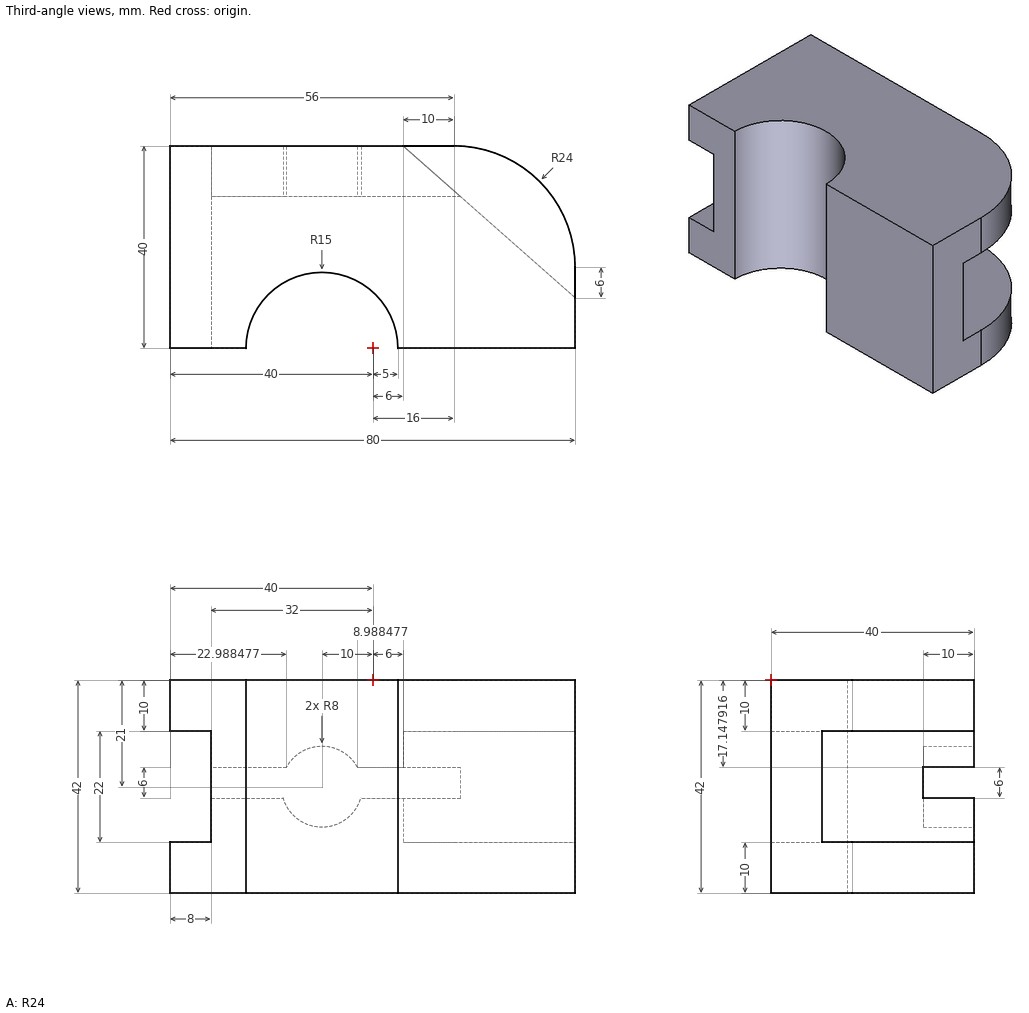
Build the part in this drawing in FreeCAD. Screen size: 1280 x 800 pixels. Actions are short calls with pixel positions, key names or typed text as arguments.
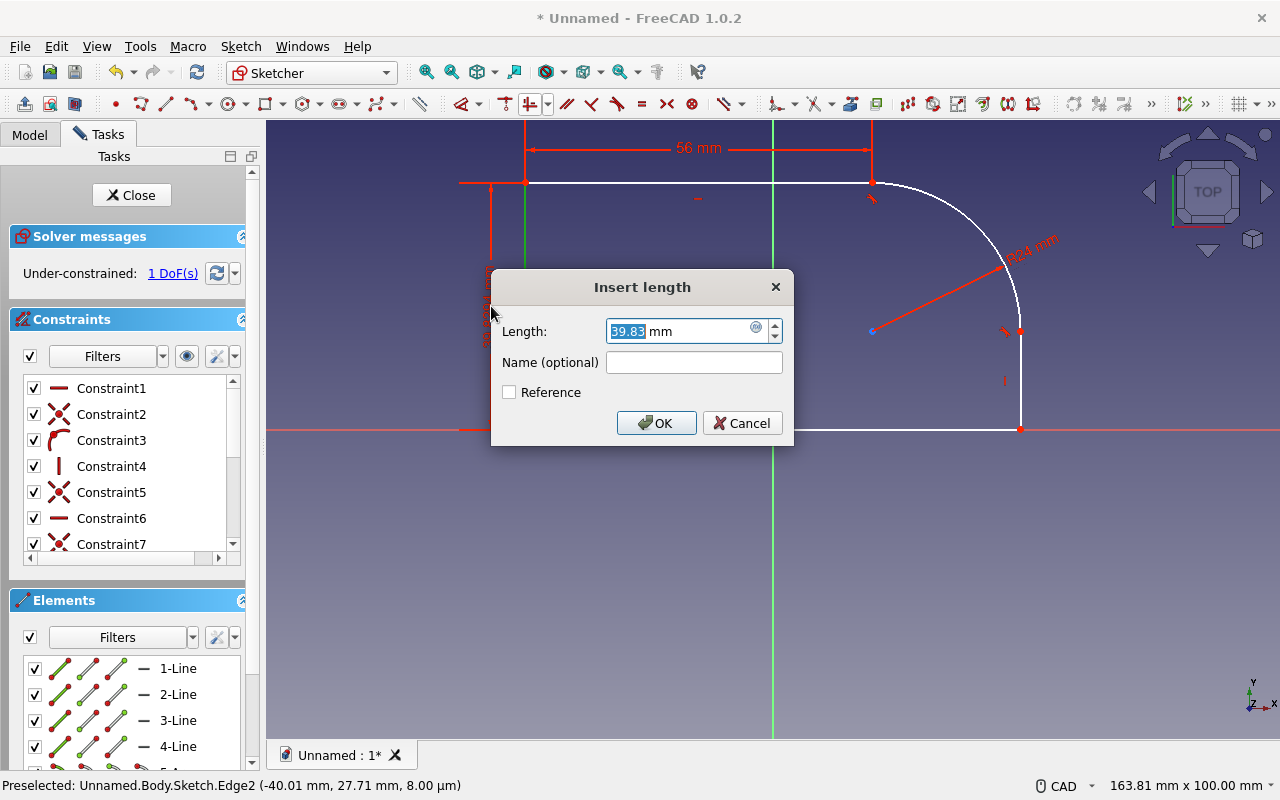
text(40)
key(Return)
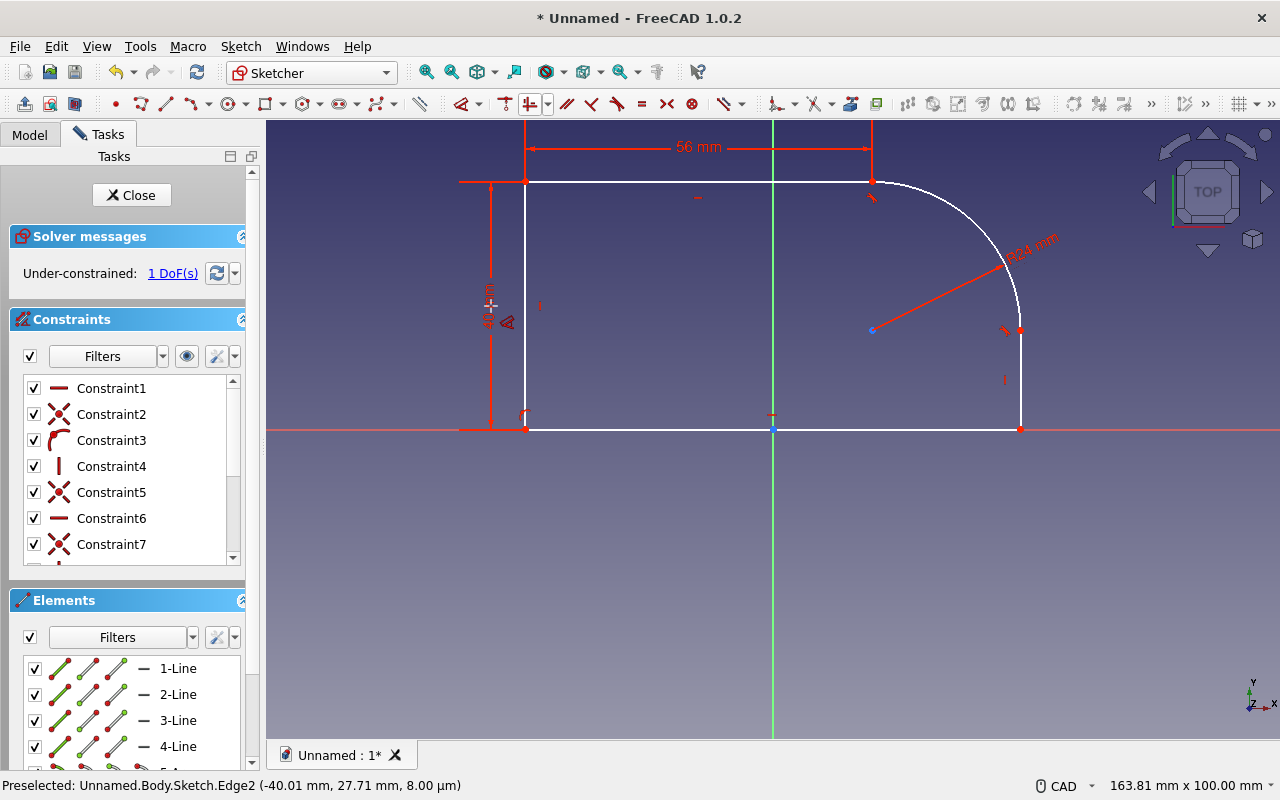
click(872, 182)
click(823, 464)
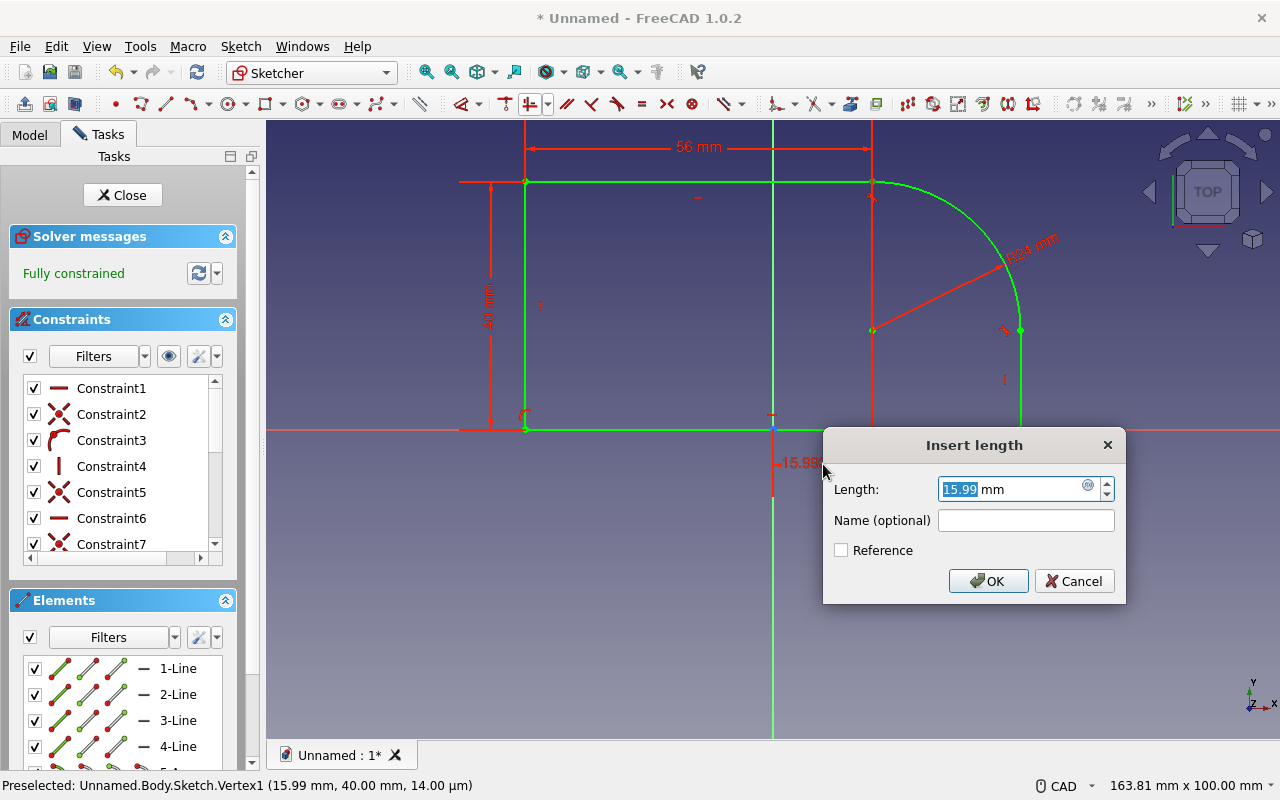
text(16)
key(Return)
key(Escape)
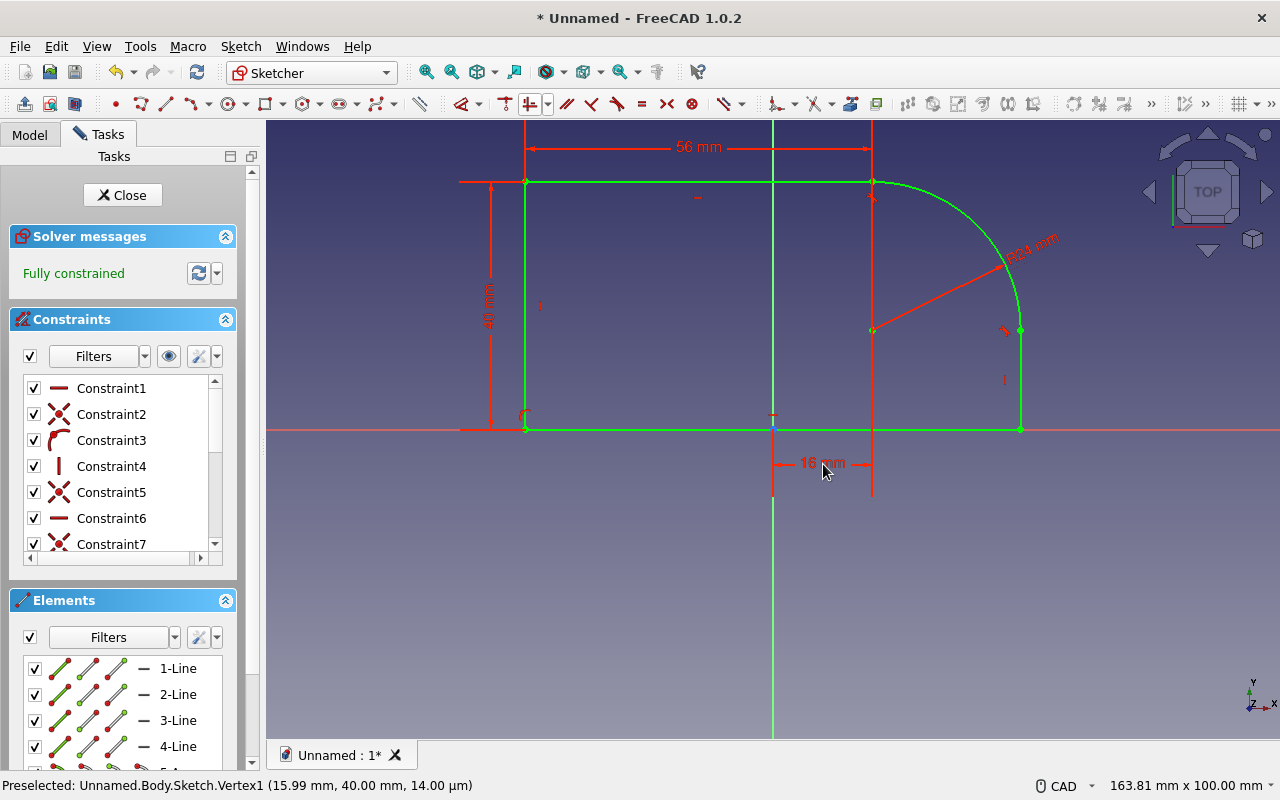
click(123, 195)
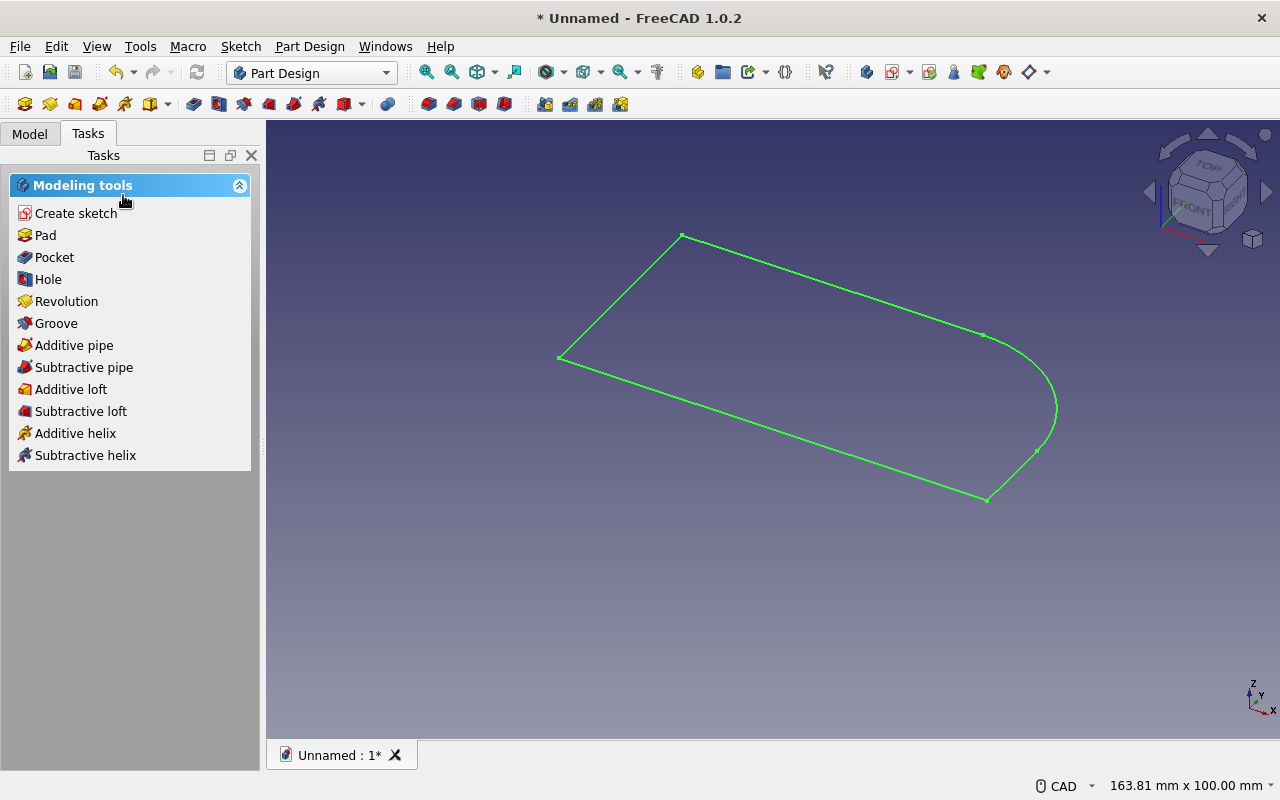
click(25, 104)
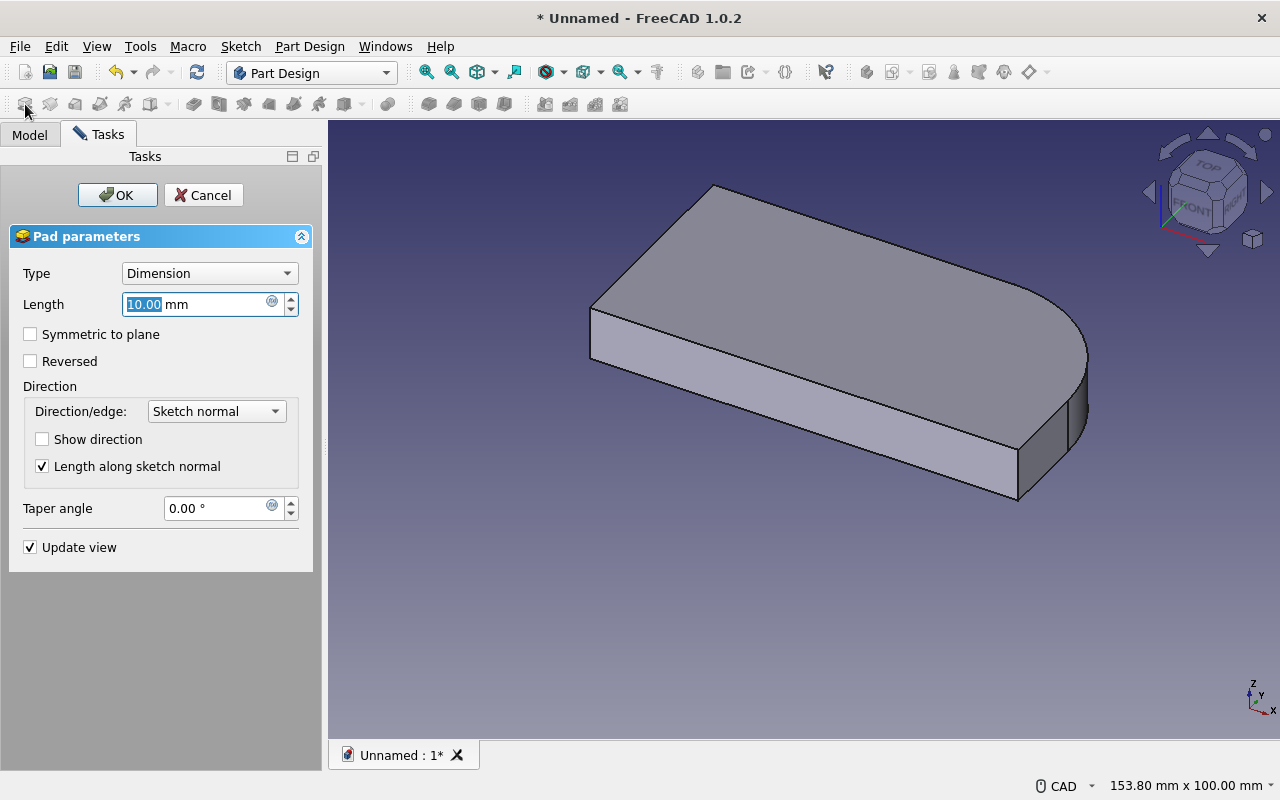
text(42)
key(Tab)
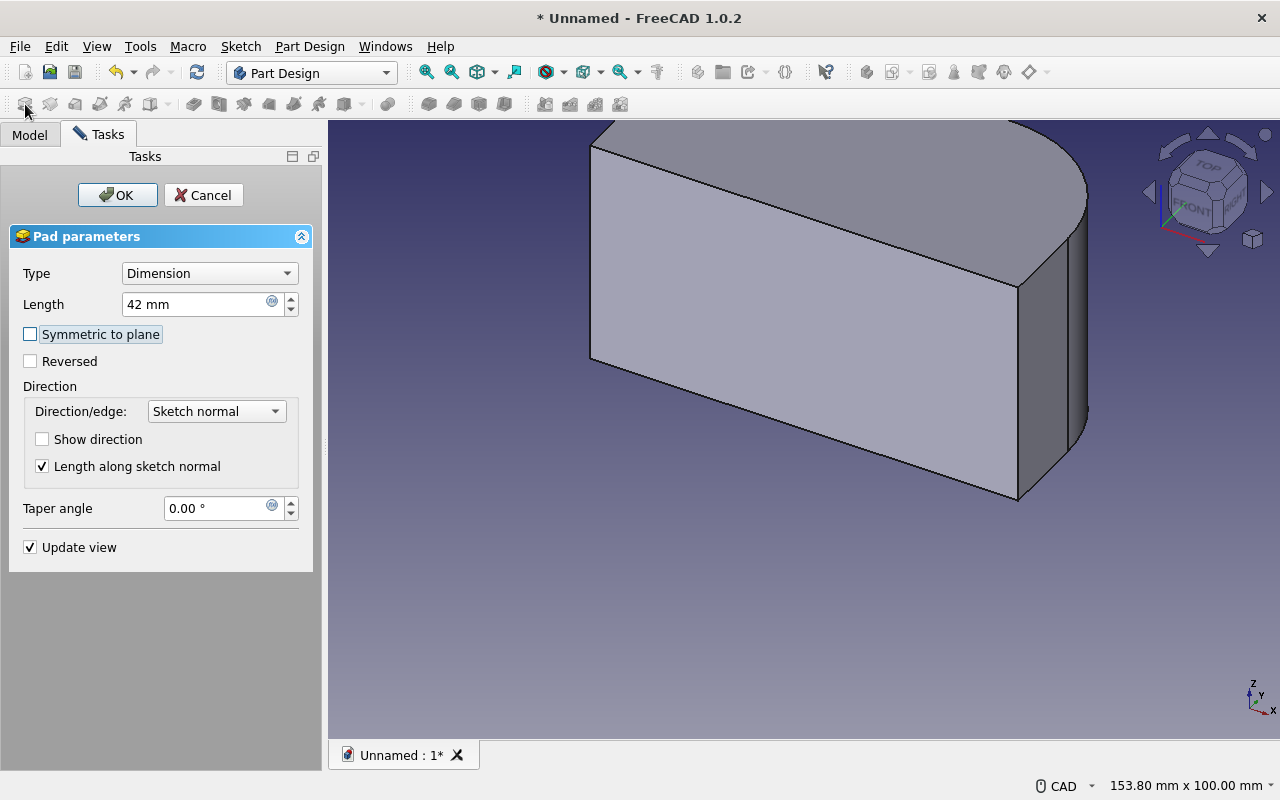
click(31, 361)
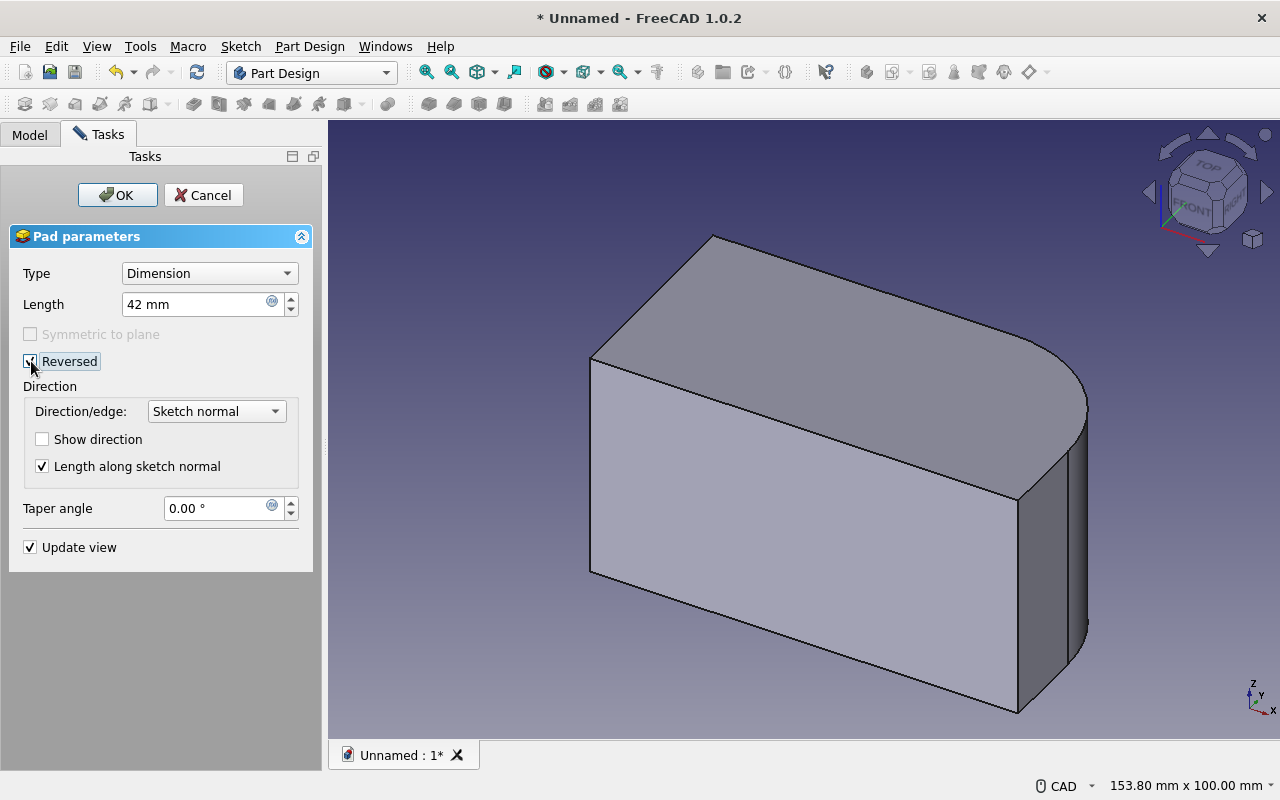
click(118, 195)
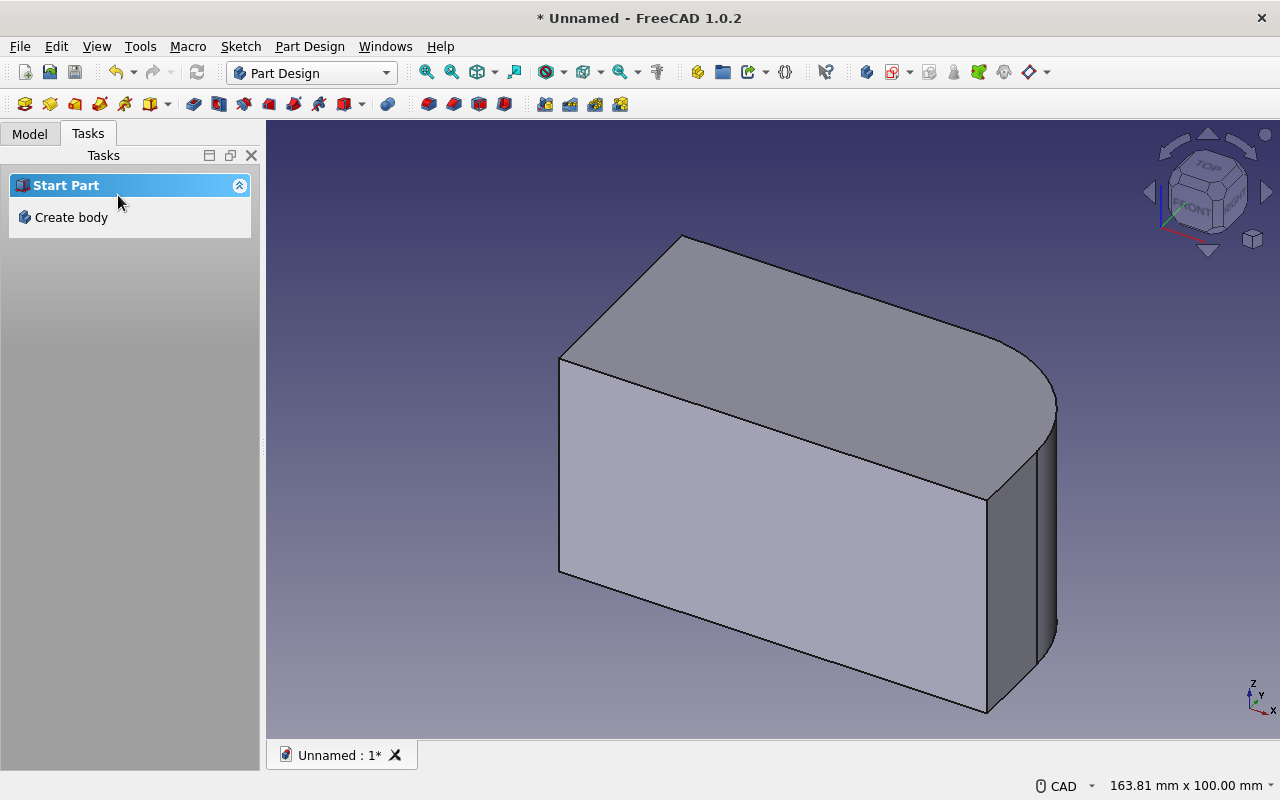
key(4)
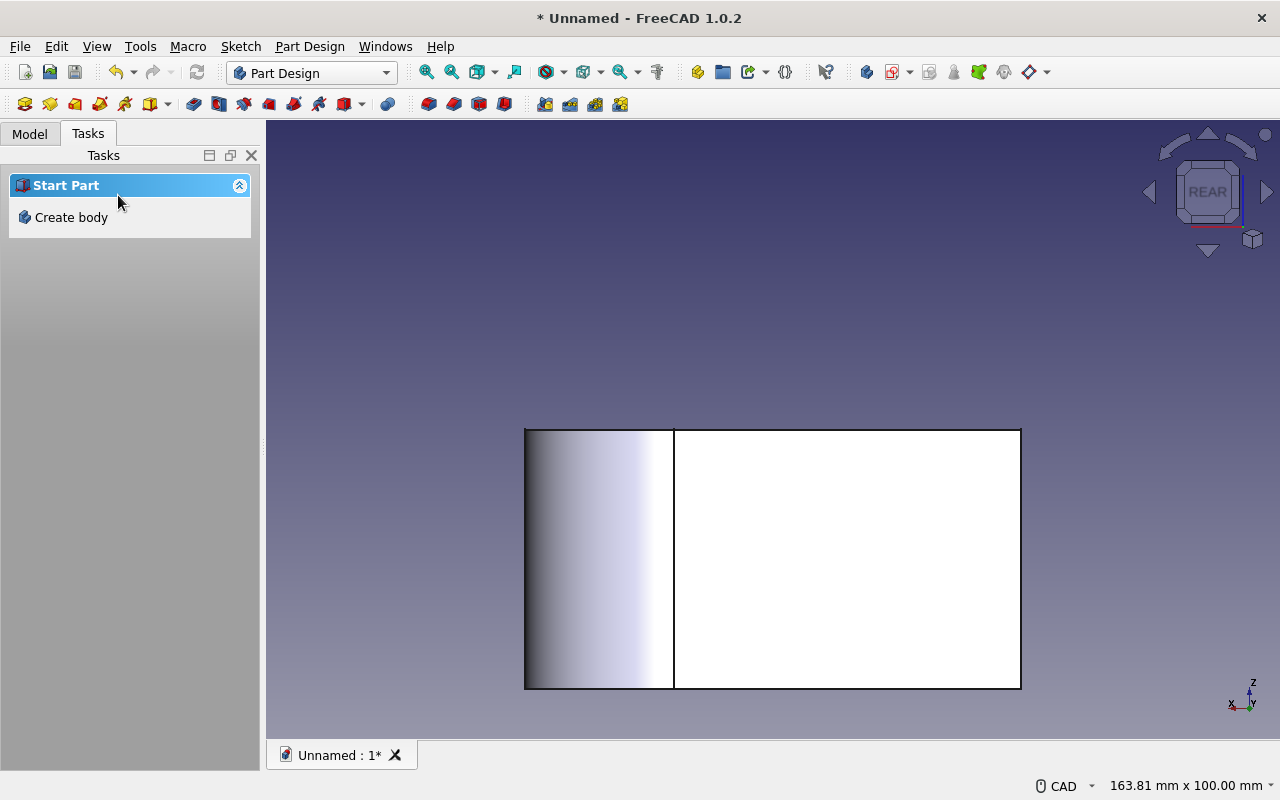
click(847, 558)